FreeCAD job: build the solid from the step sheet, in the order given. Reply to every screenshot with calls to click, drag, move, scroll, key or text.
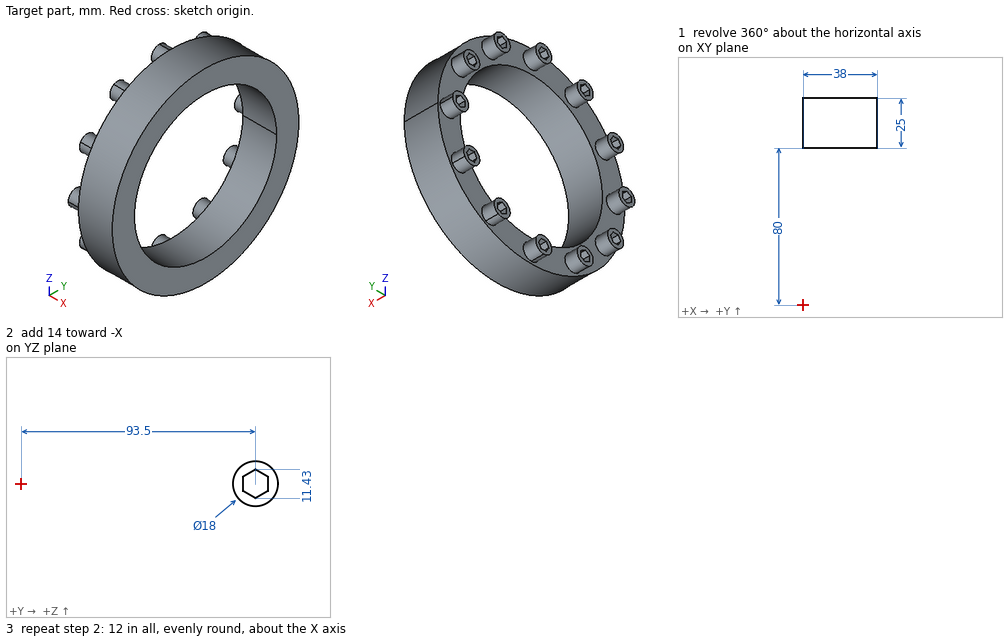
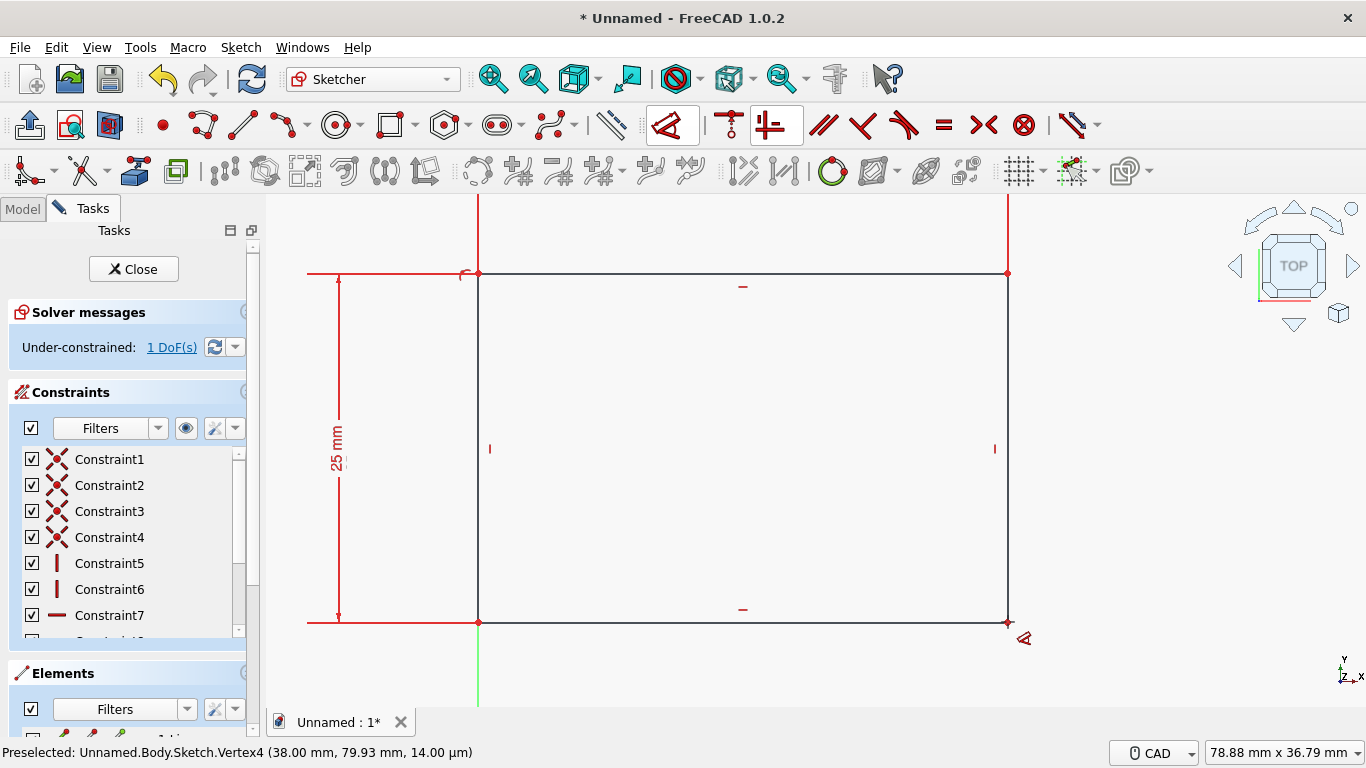
click(478, 623)
click(444, 651)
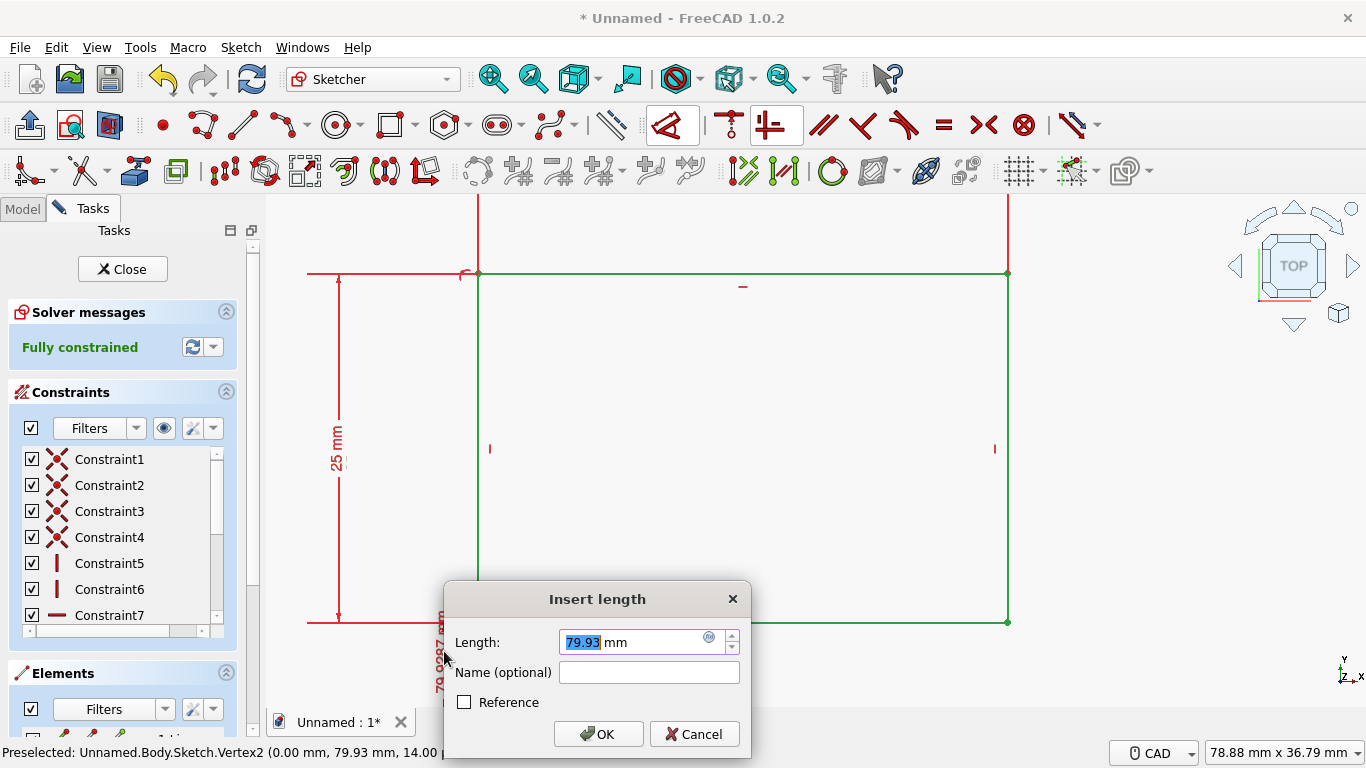
text(80)
key(Return)
key(Escape)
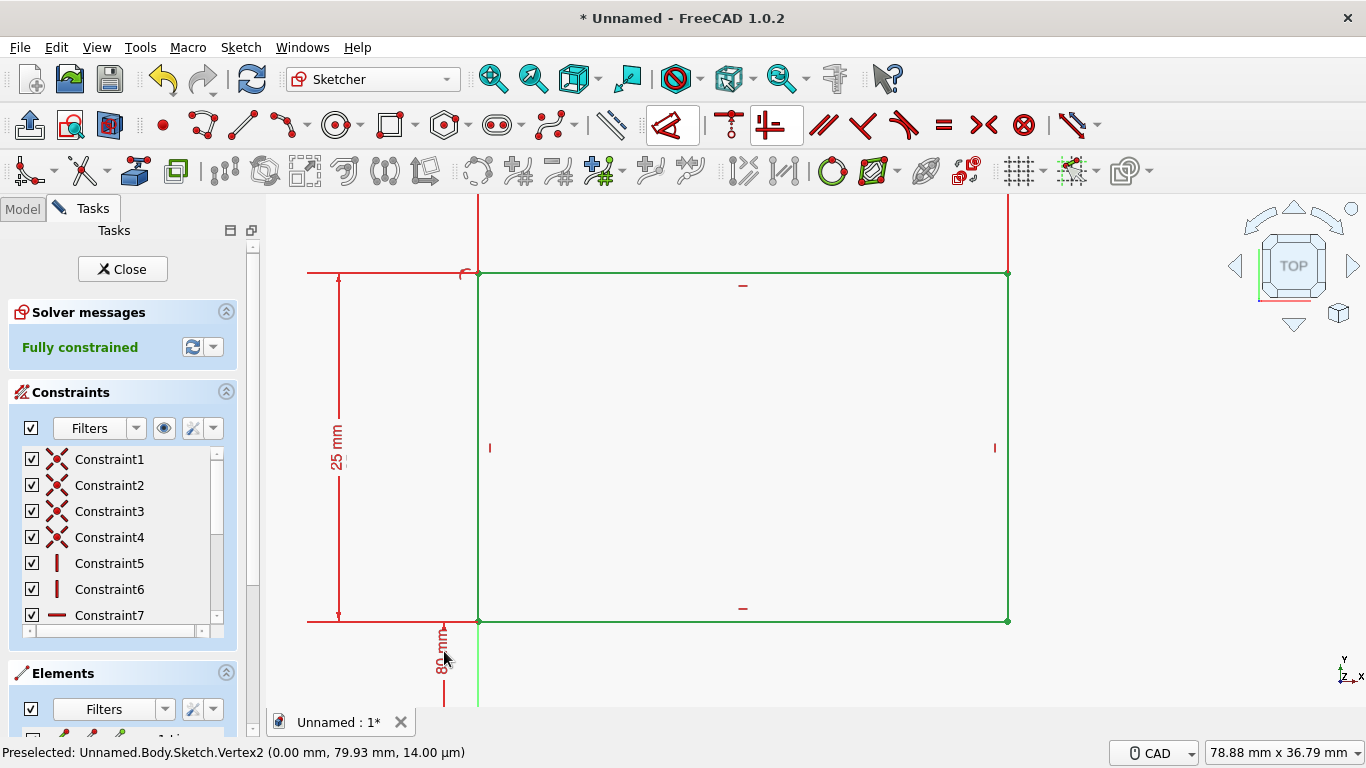
click(123, 269)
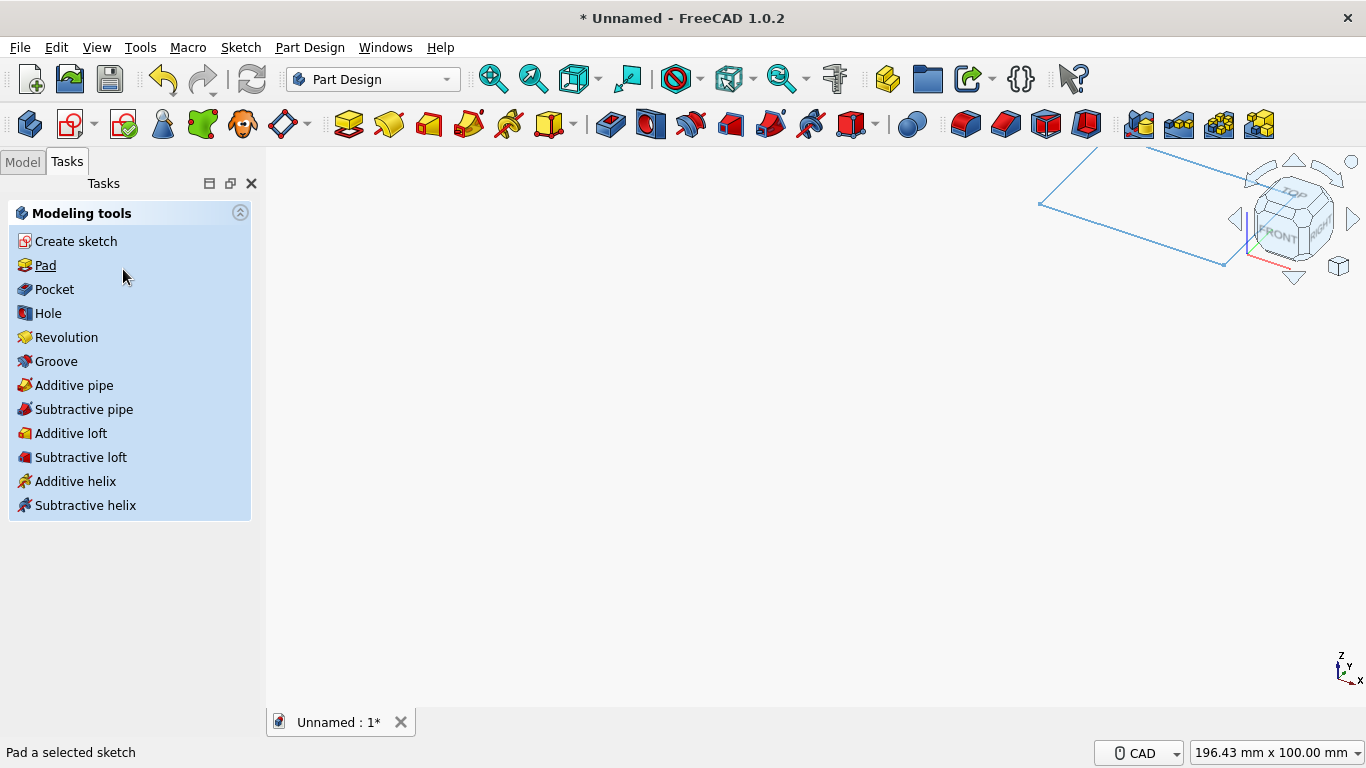
click(390, 124)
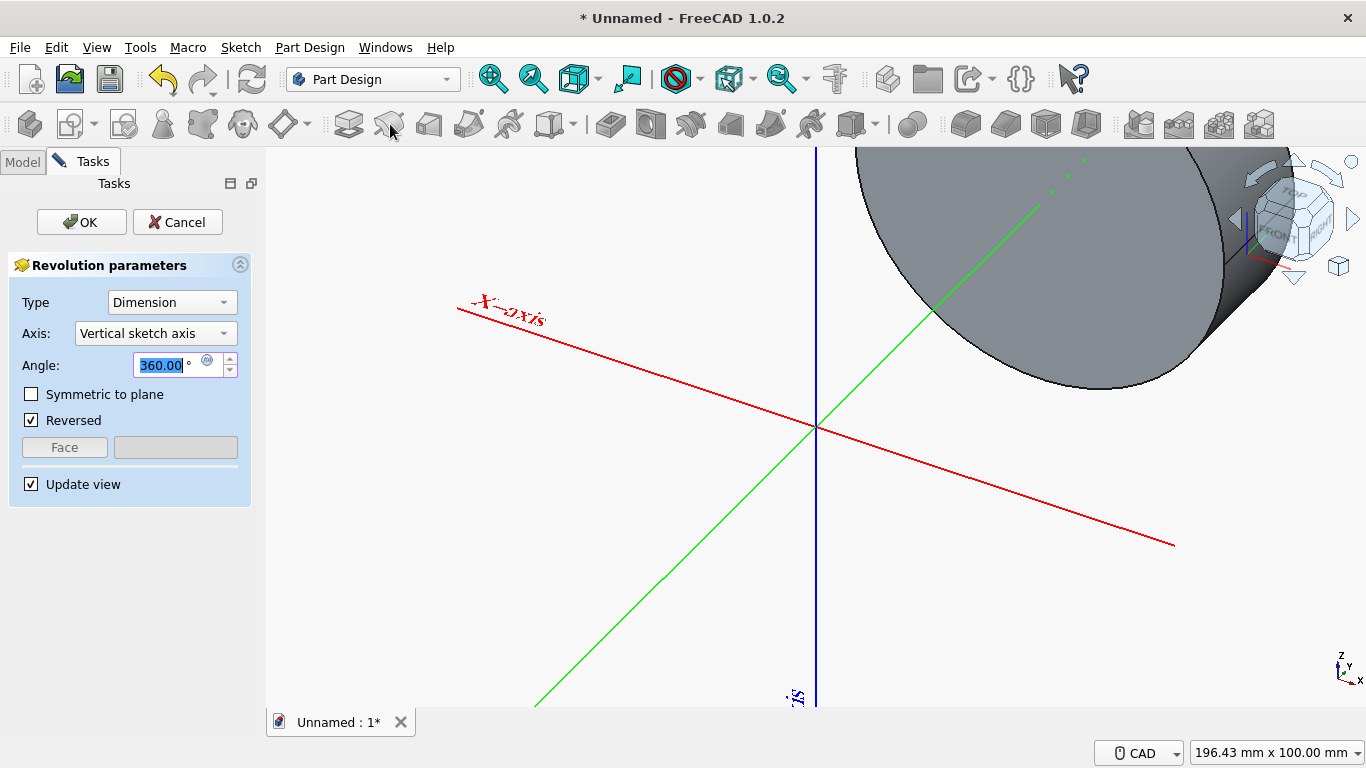
click(156, 334)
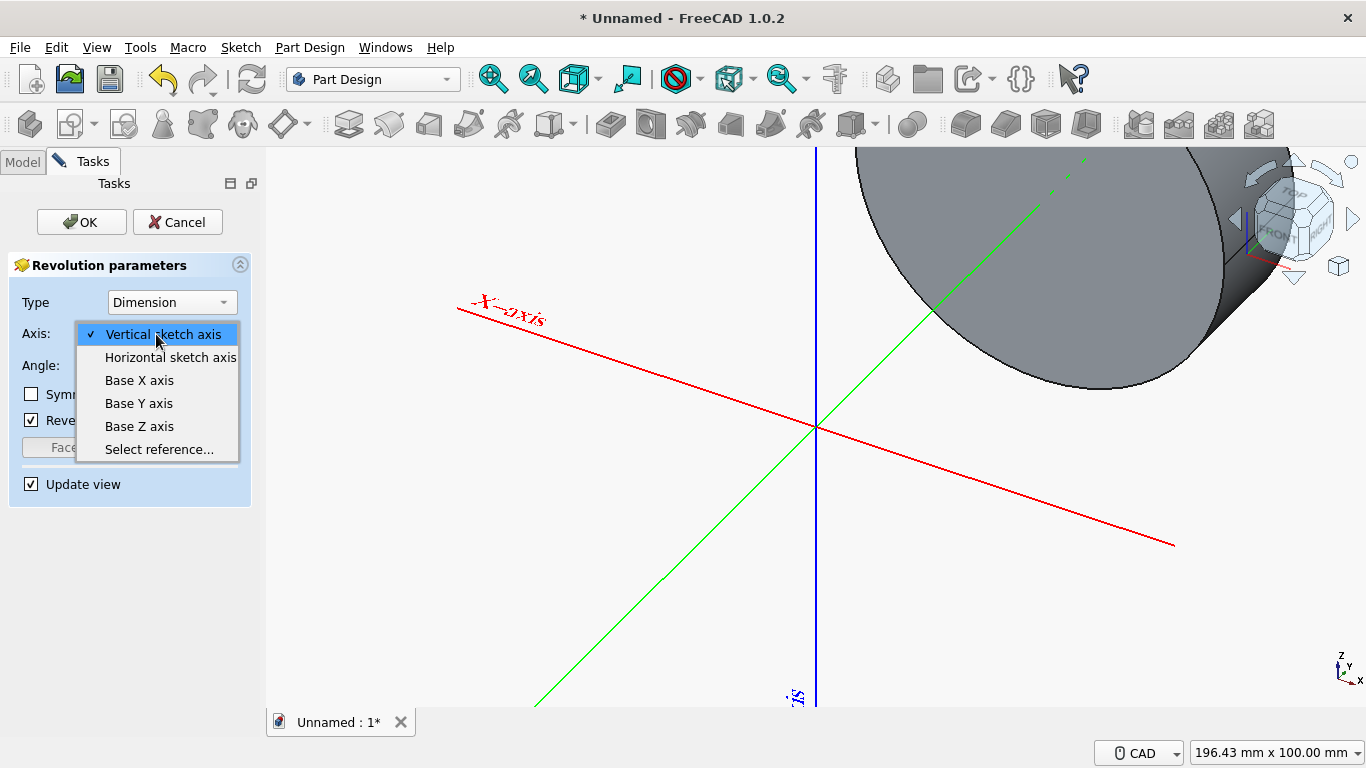
click(156, 358)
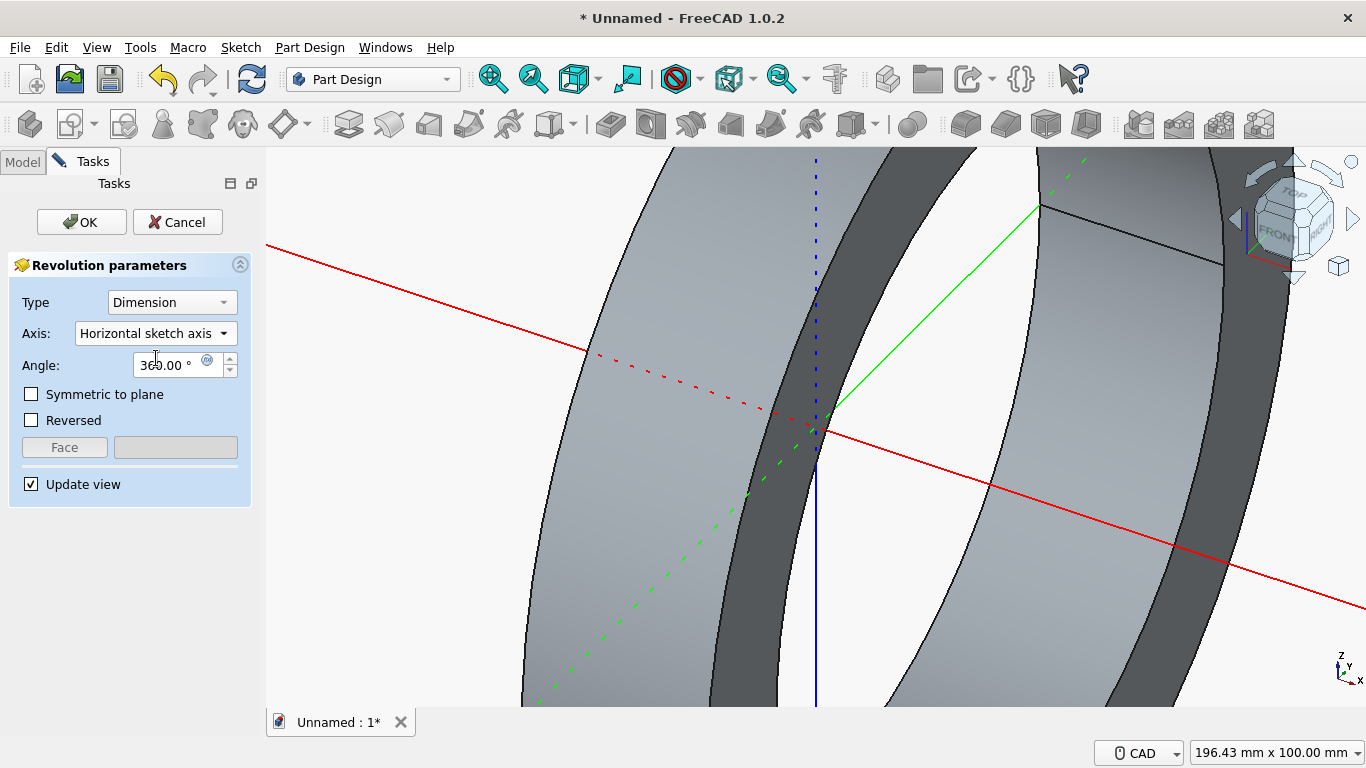
click(82, 222)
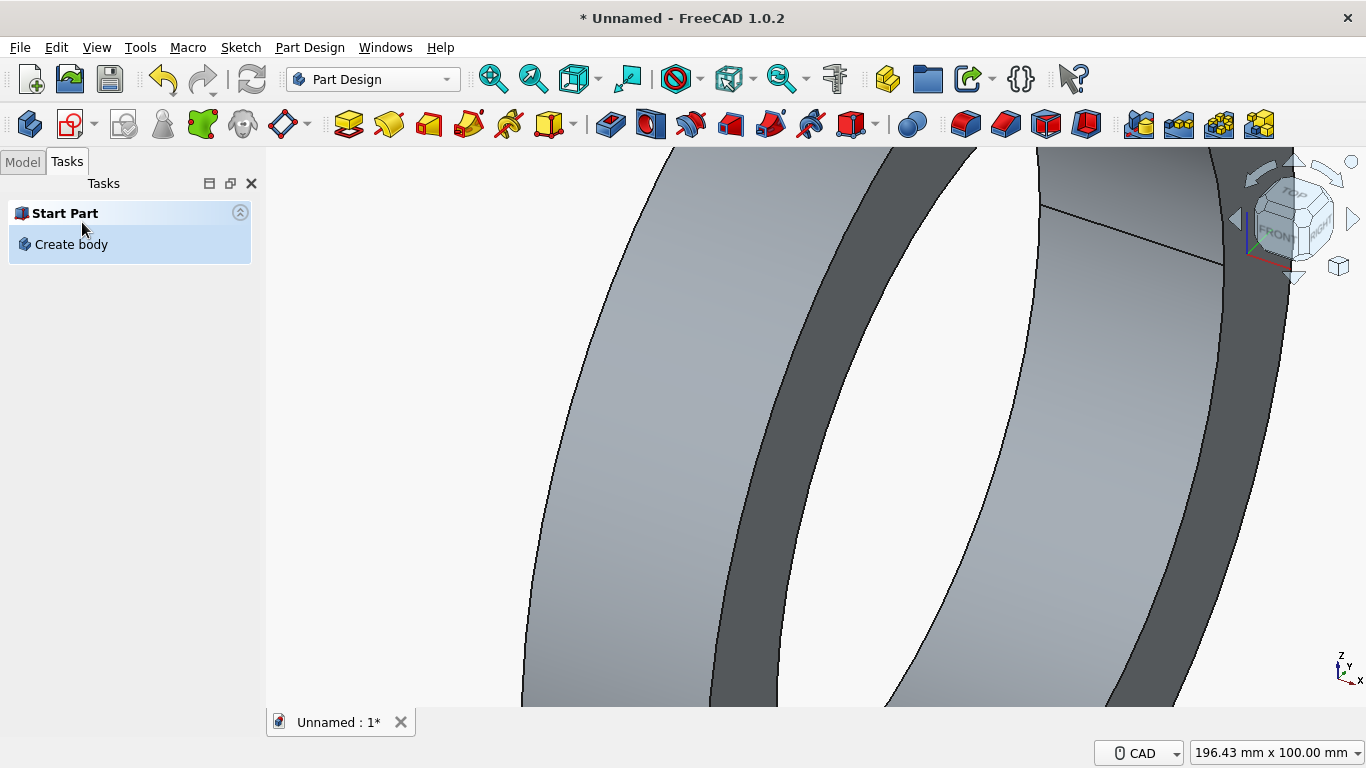
click(494, 80)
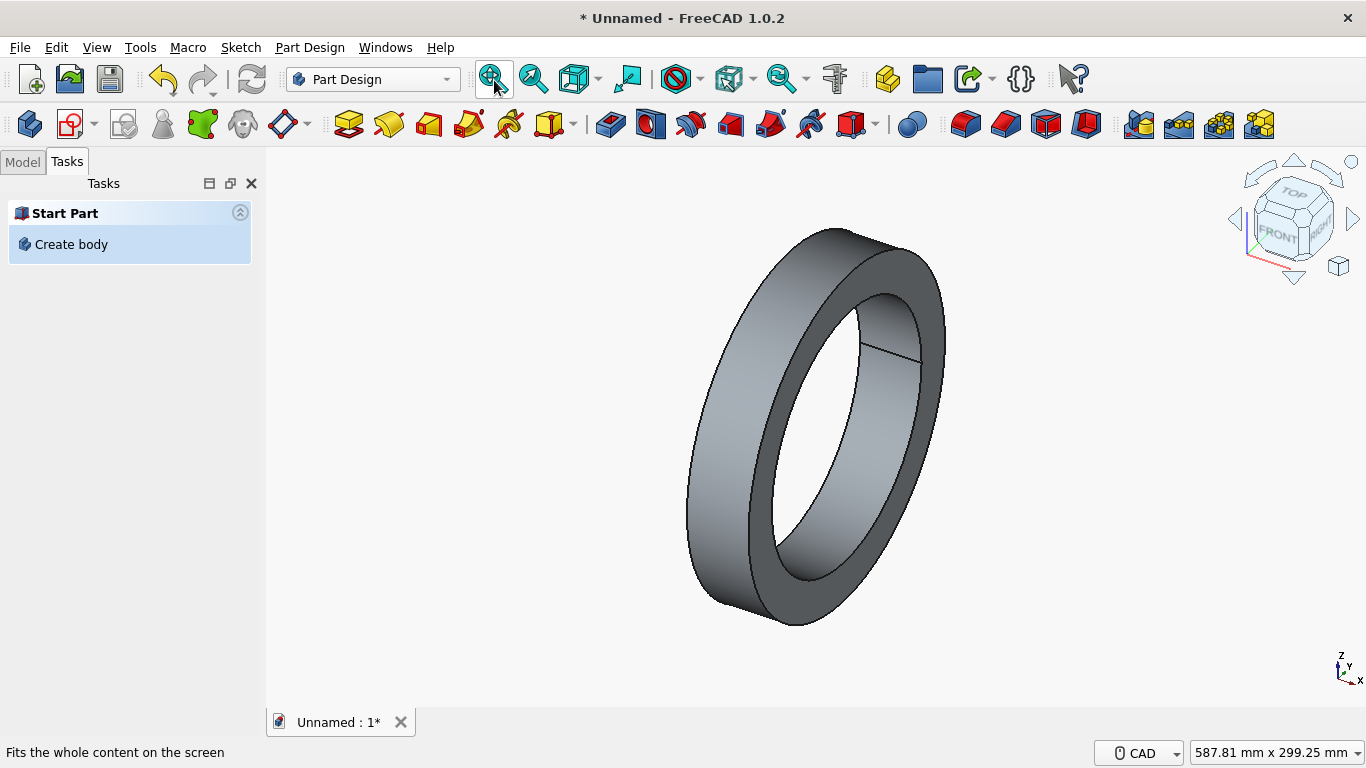
click(70, 124)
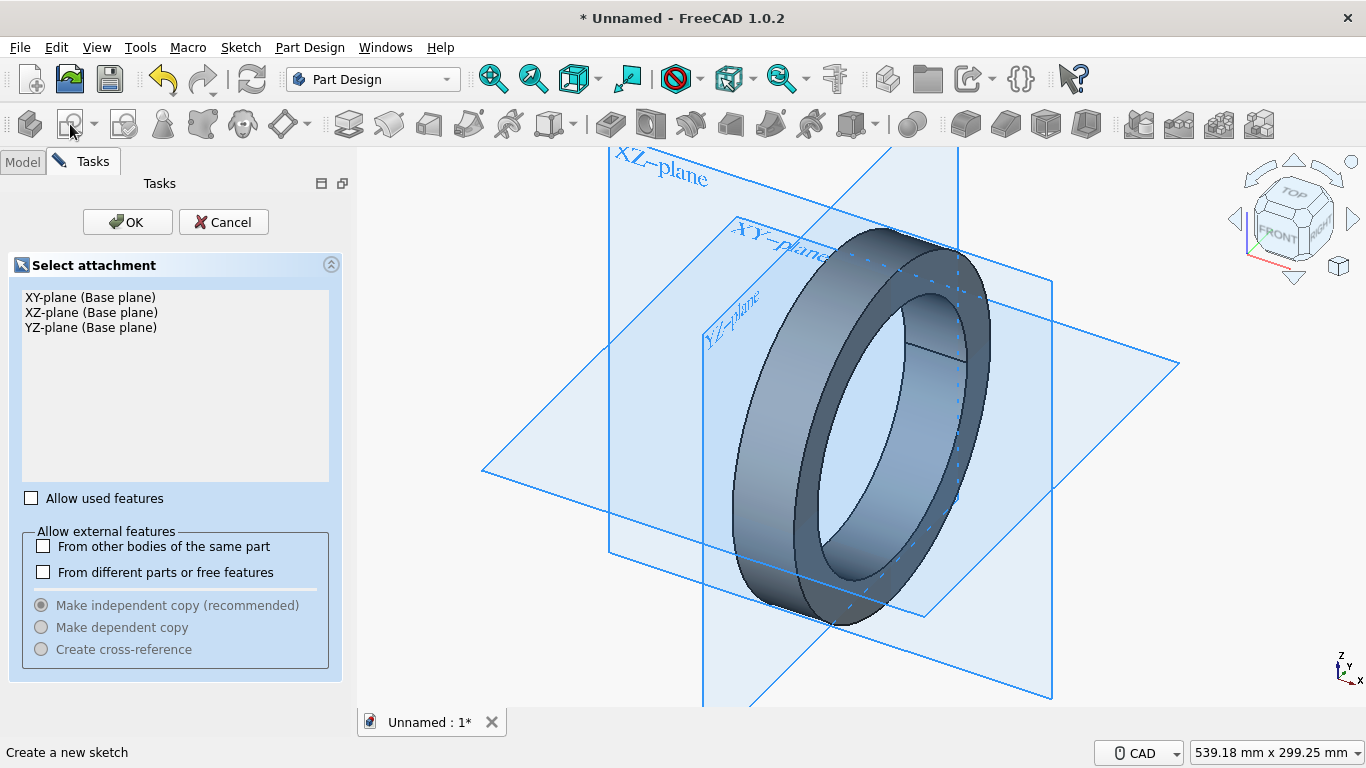
click(82, 328)